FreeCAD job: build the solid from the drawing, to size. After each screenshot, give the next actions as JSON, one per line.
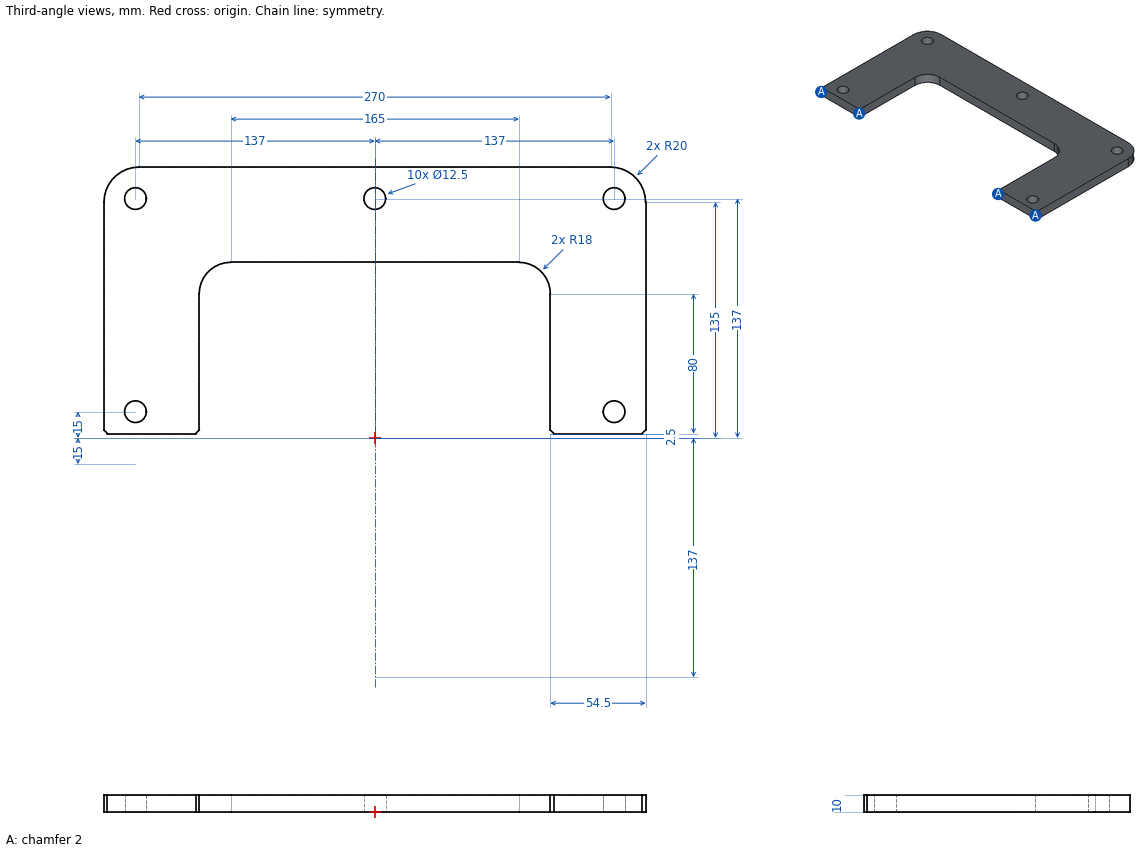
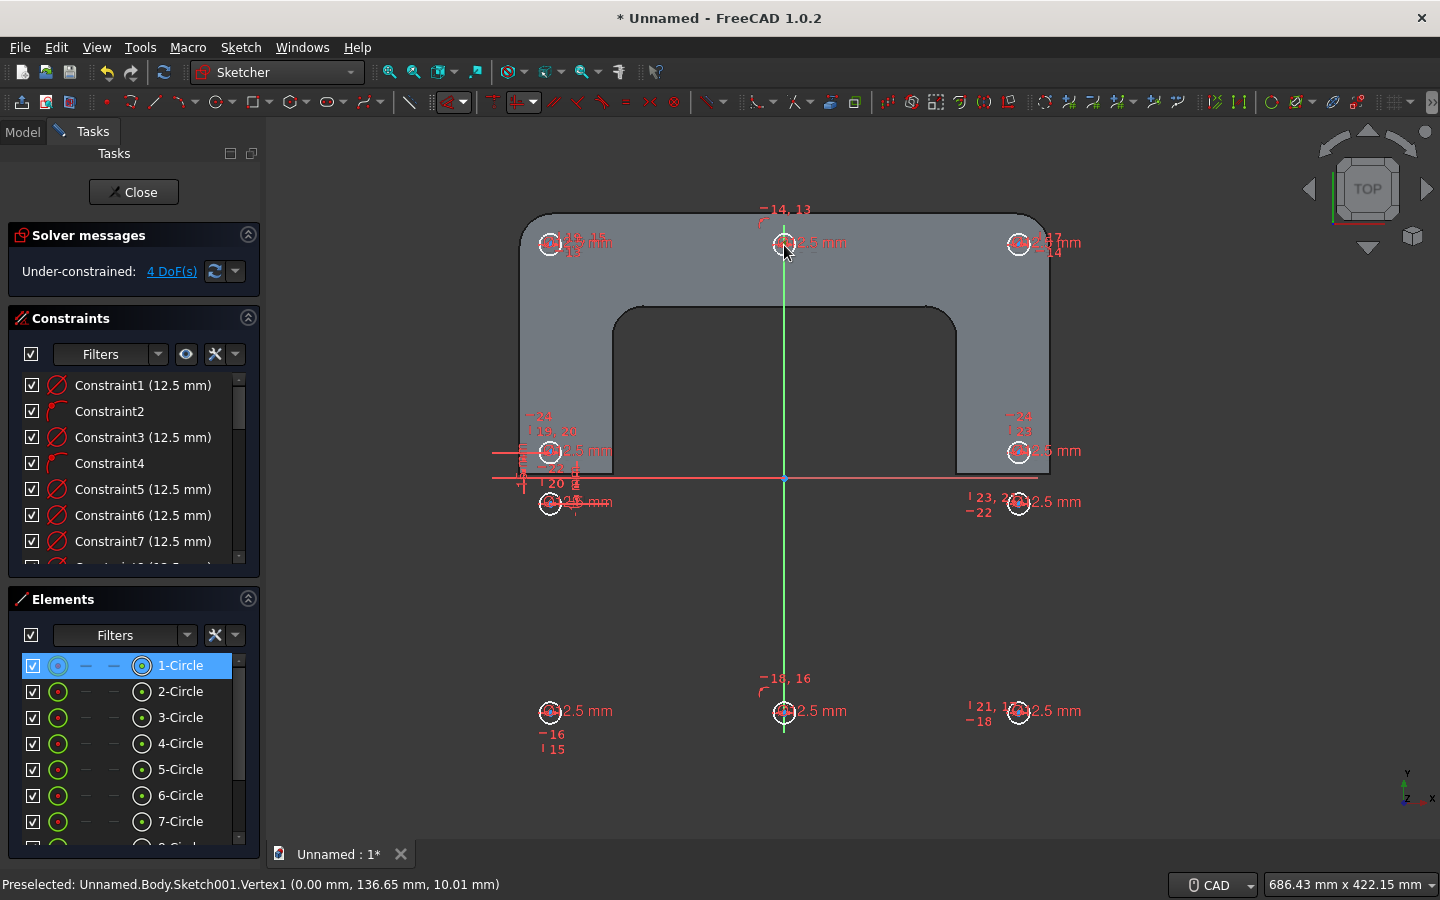
{"action": "key", "text": "i"}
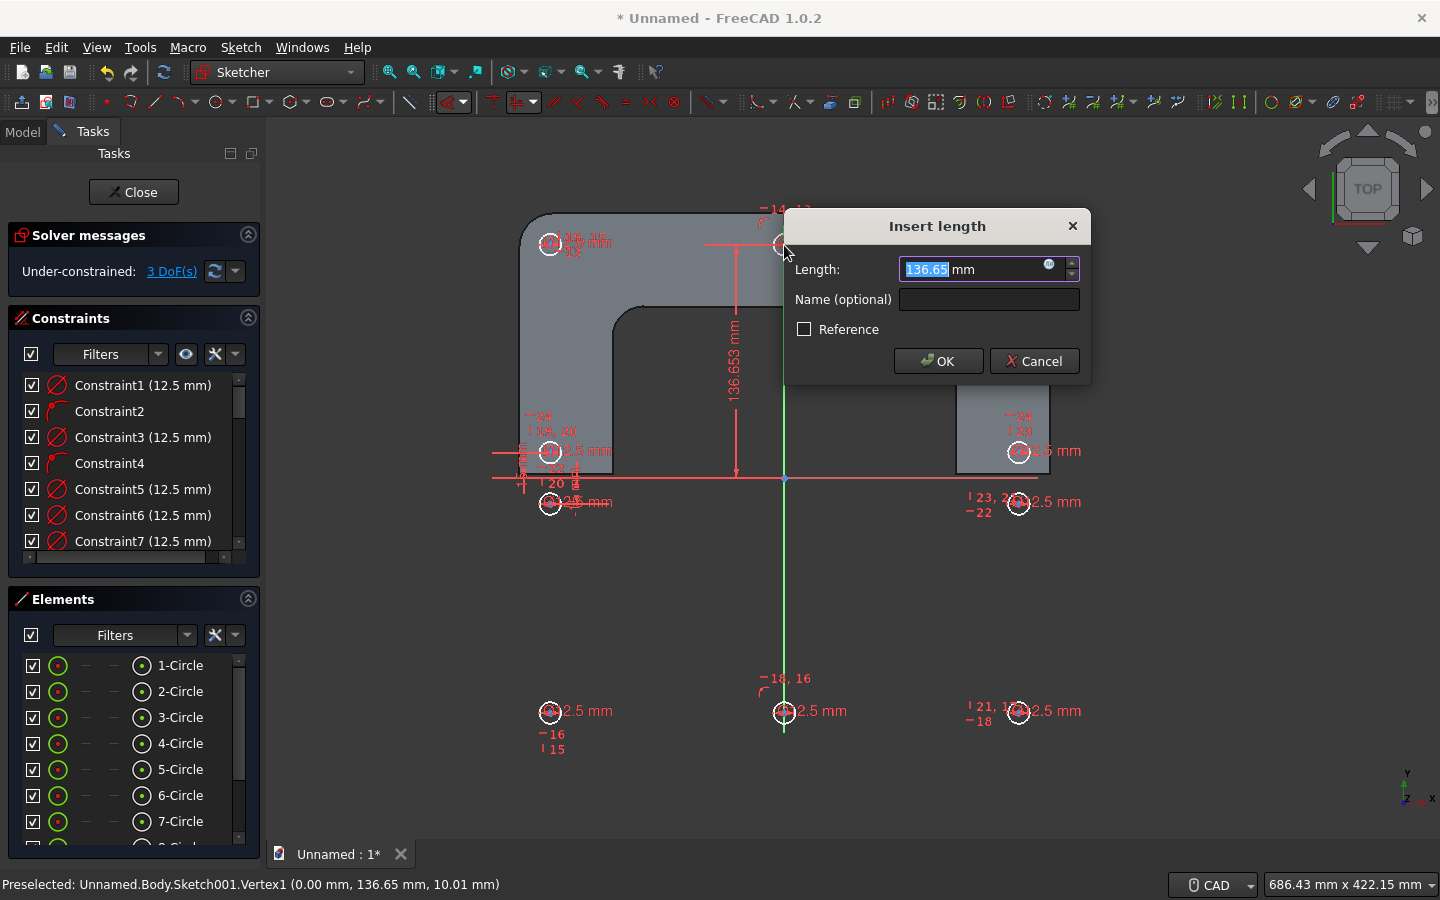
{"action": "type", "text": "137"}
{"action": "key", "text": "Return"}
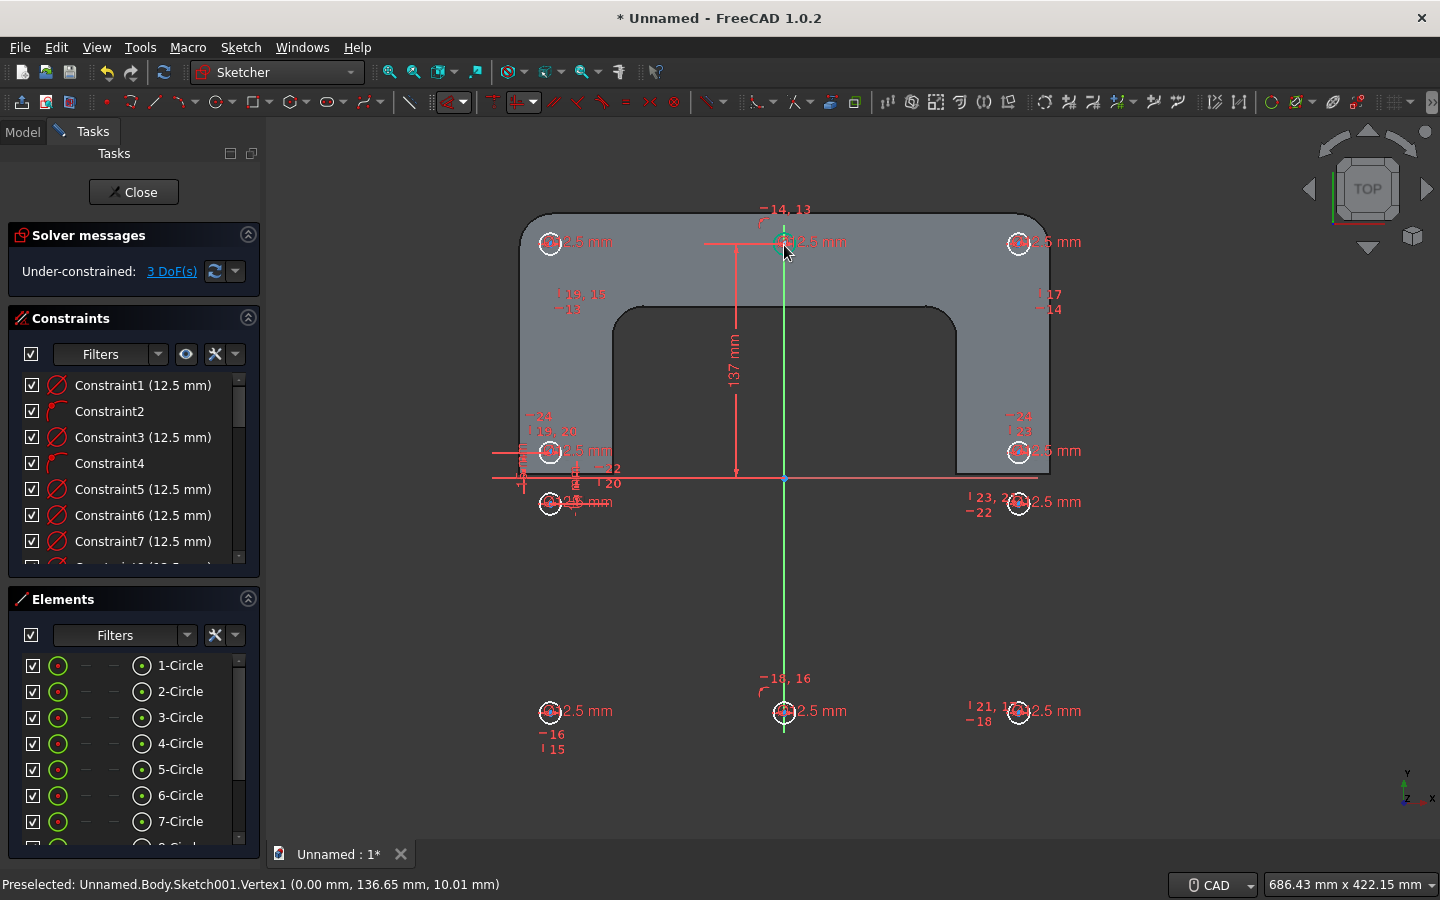
{"action": "left_click", "coordinate": [784, 713]}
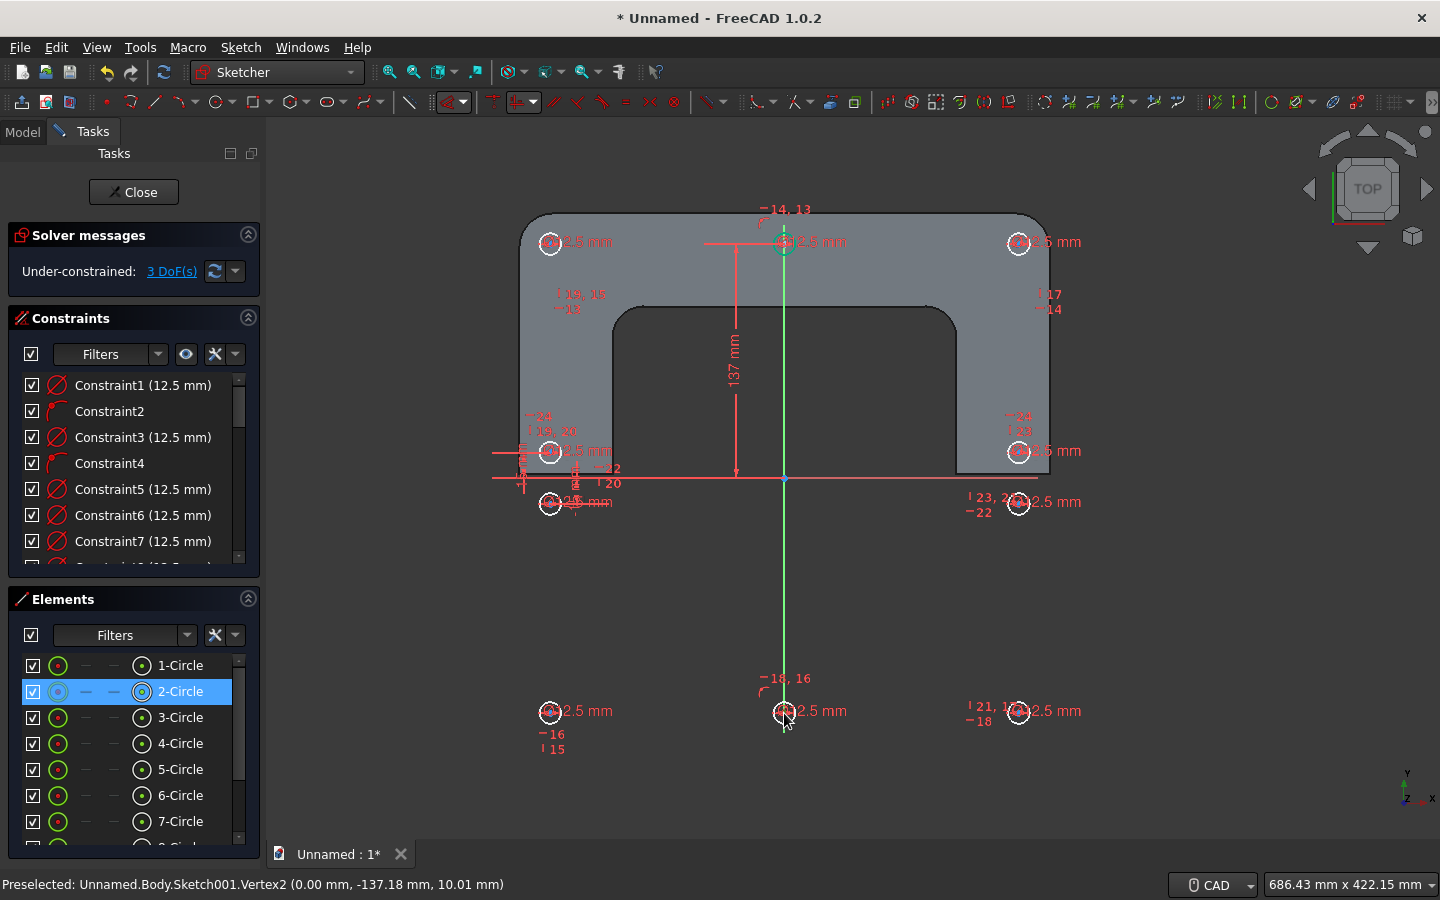
{"action": "key", "text": "i"}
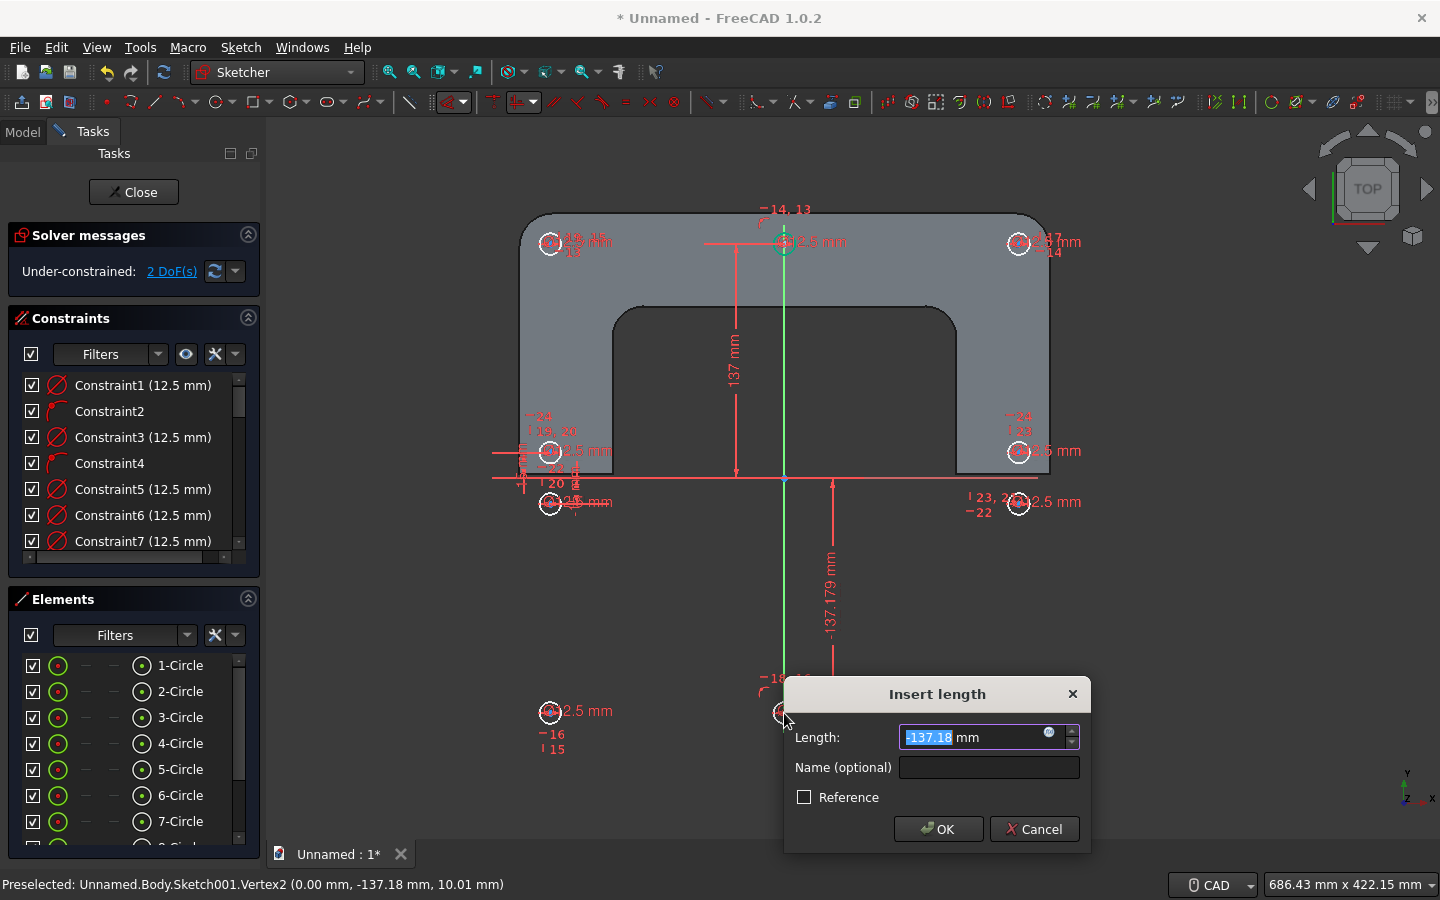
{"action": "type", "text": "-137"}
{"action": "key", "text": "Return"}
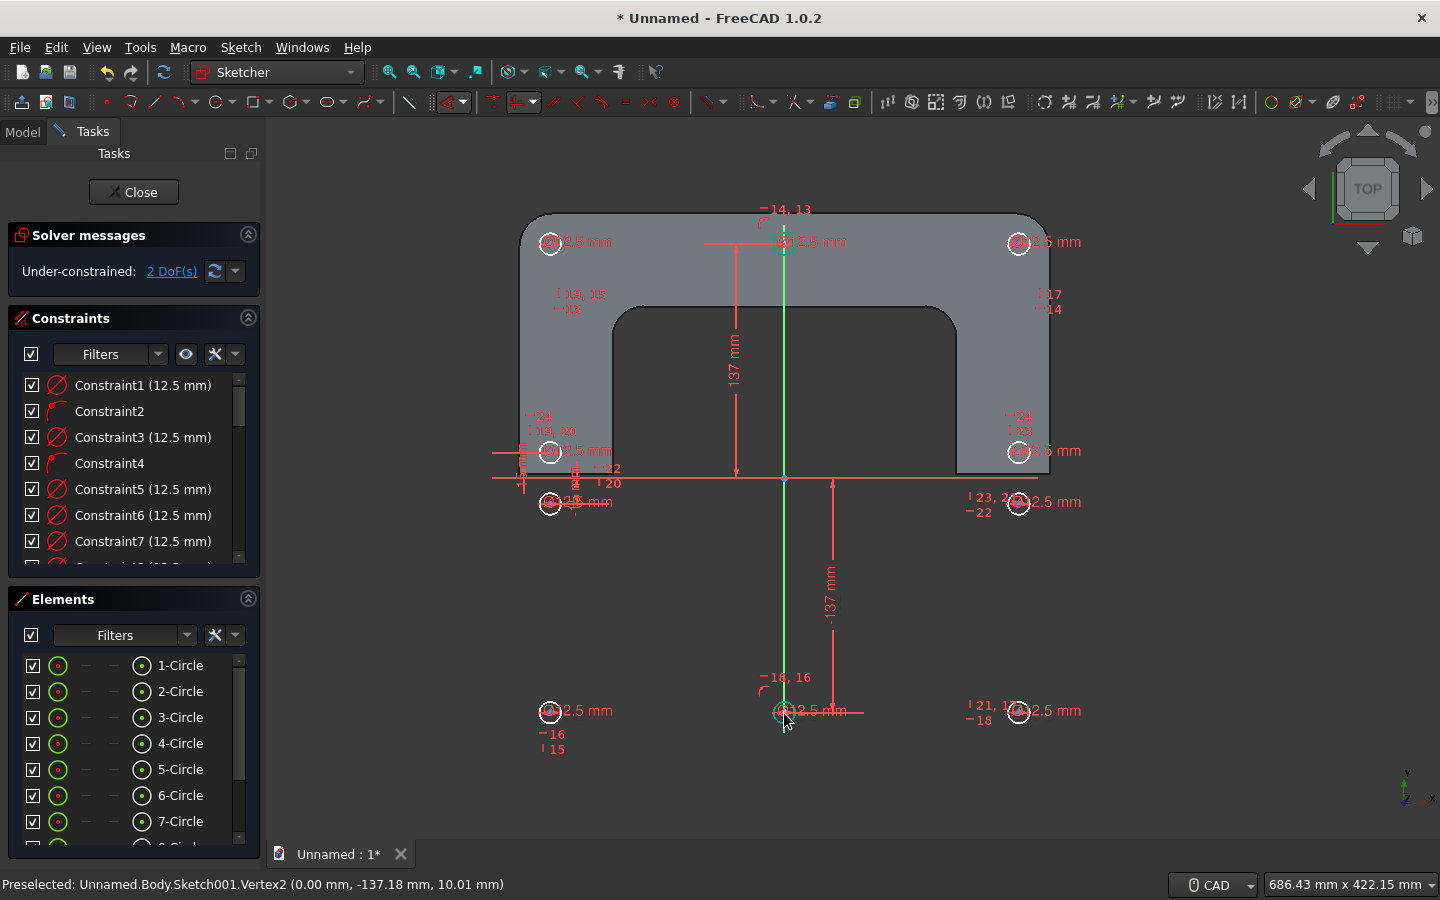
{"action": "left_click", "coordinate": [550, 244]}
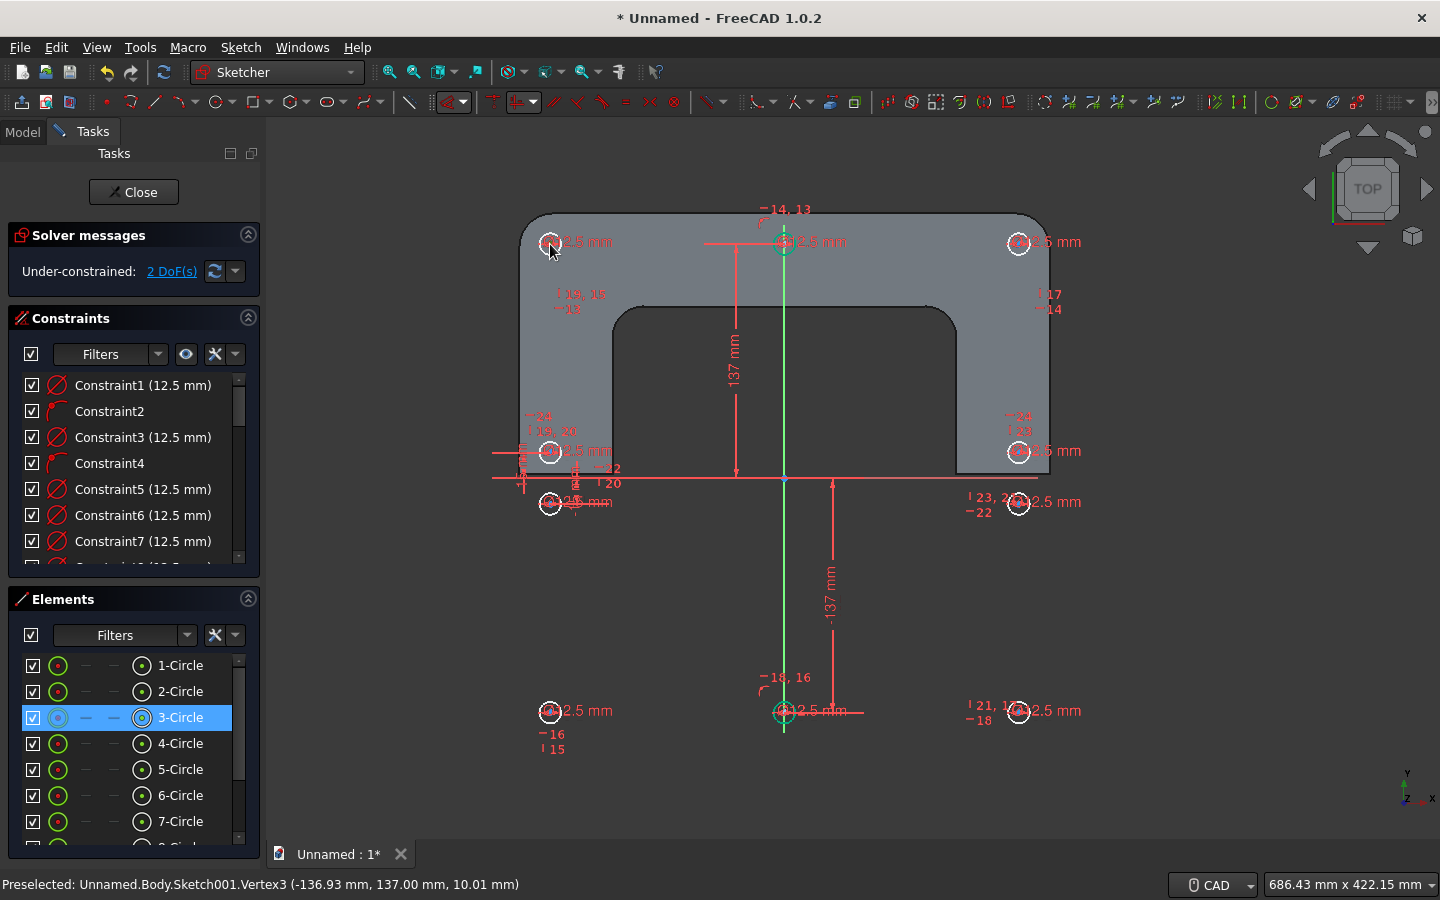
{"action": "key", "text": "l"}